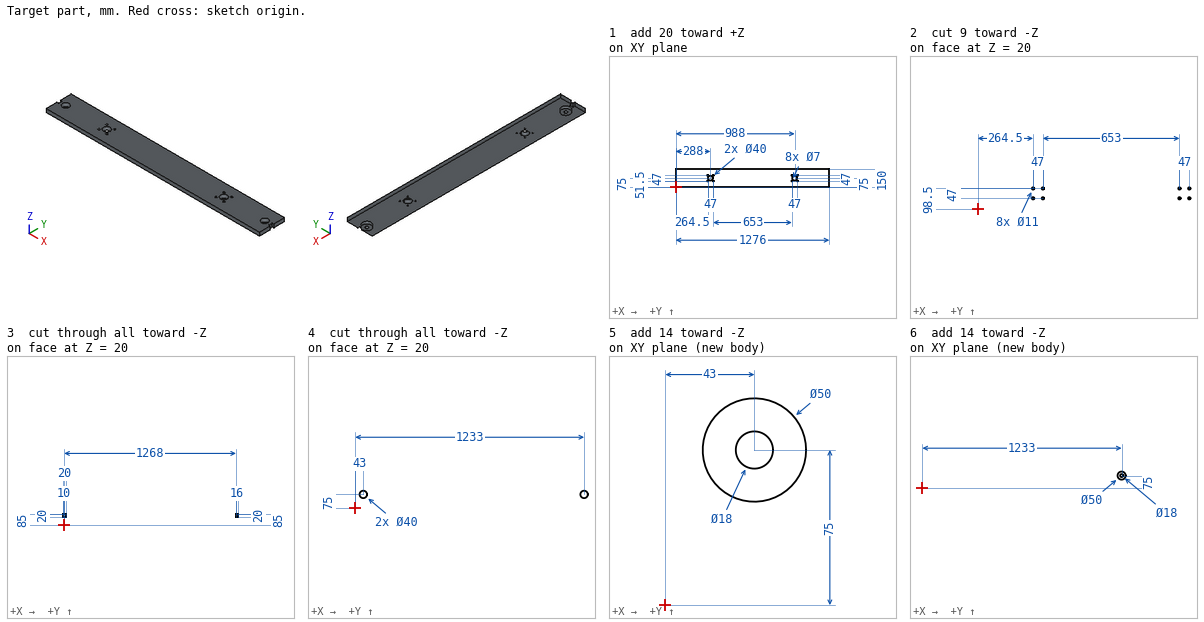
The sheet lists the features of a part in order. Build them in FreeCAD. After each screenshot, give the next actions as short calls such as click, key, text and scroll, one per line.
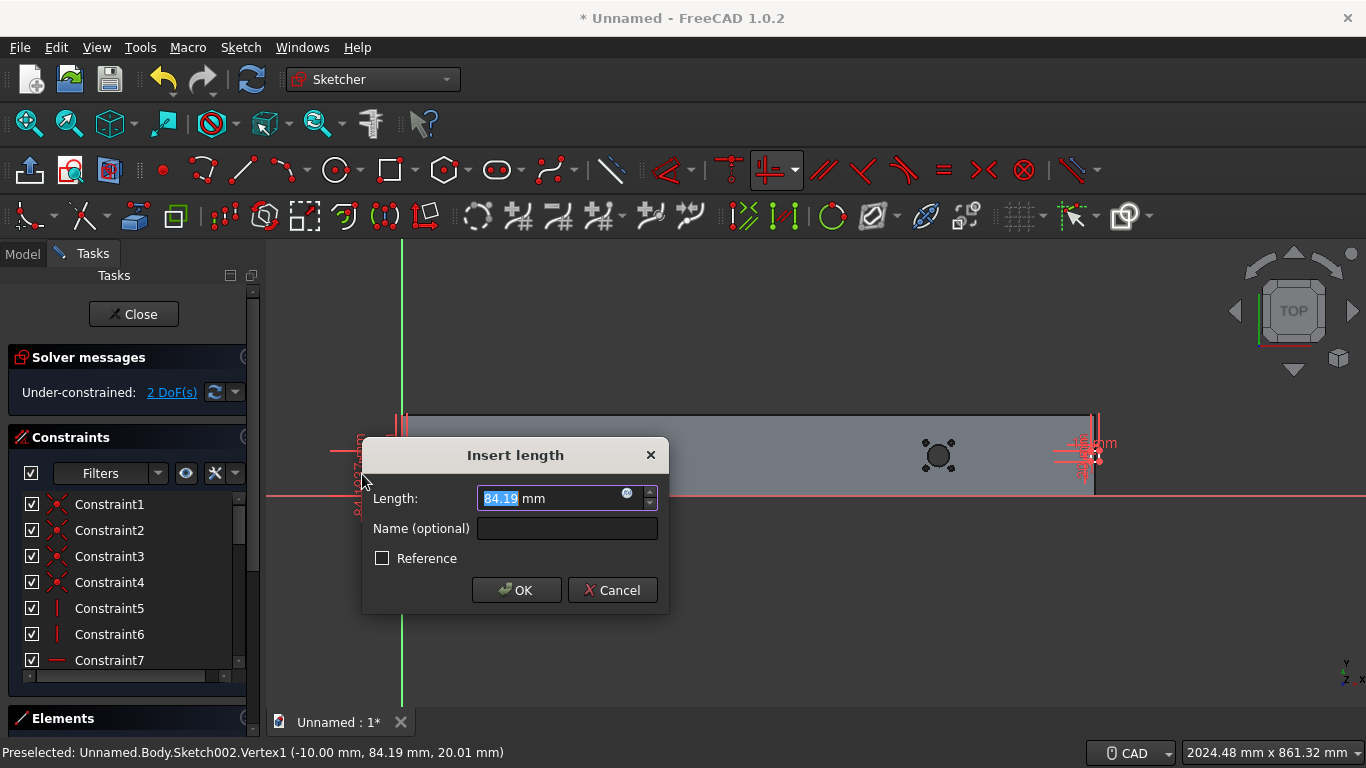
text(85)
key(Return)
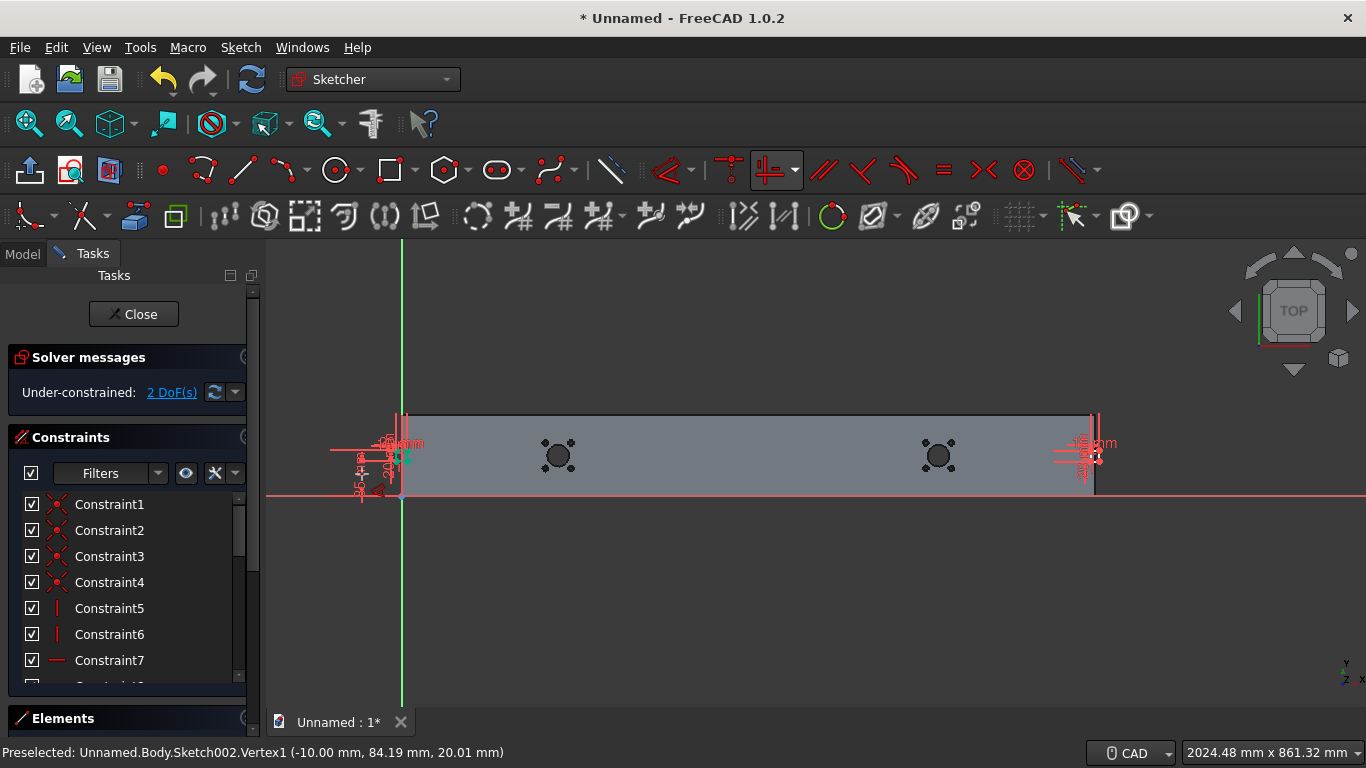
scroll(1091, 451, up, 2)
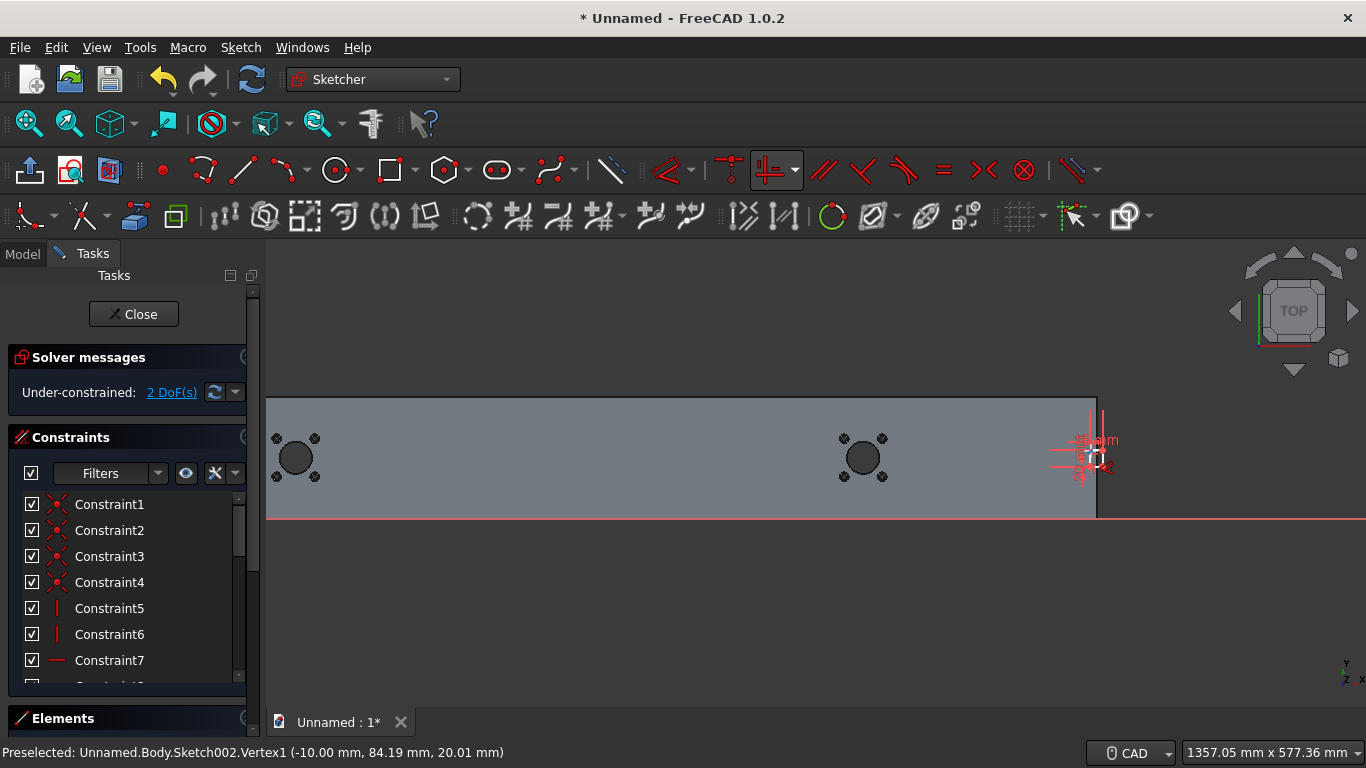
click(1090, 450)
click(1124, 484)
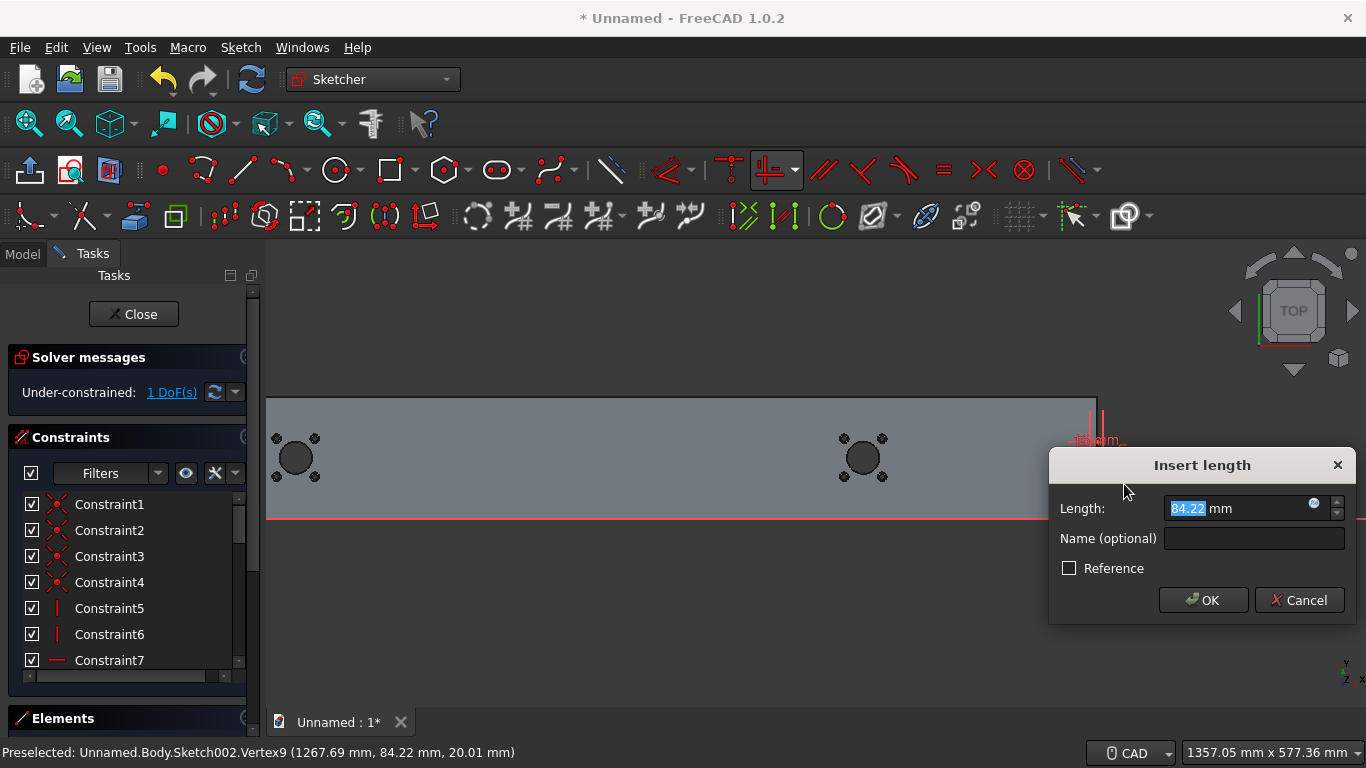
text(85)
key(Return)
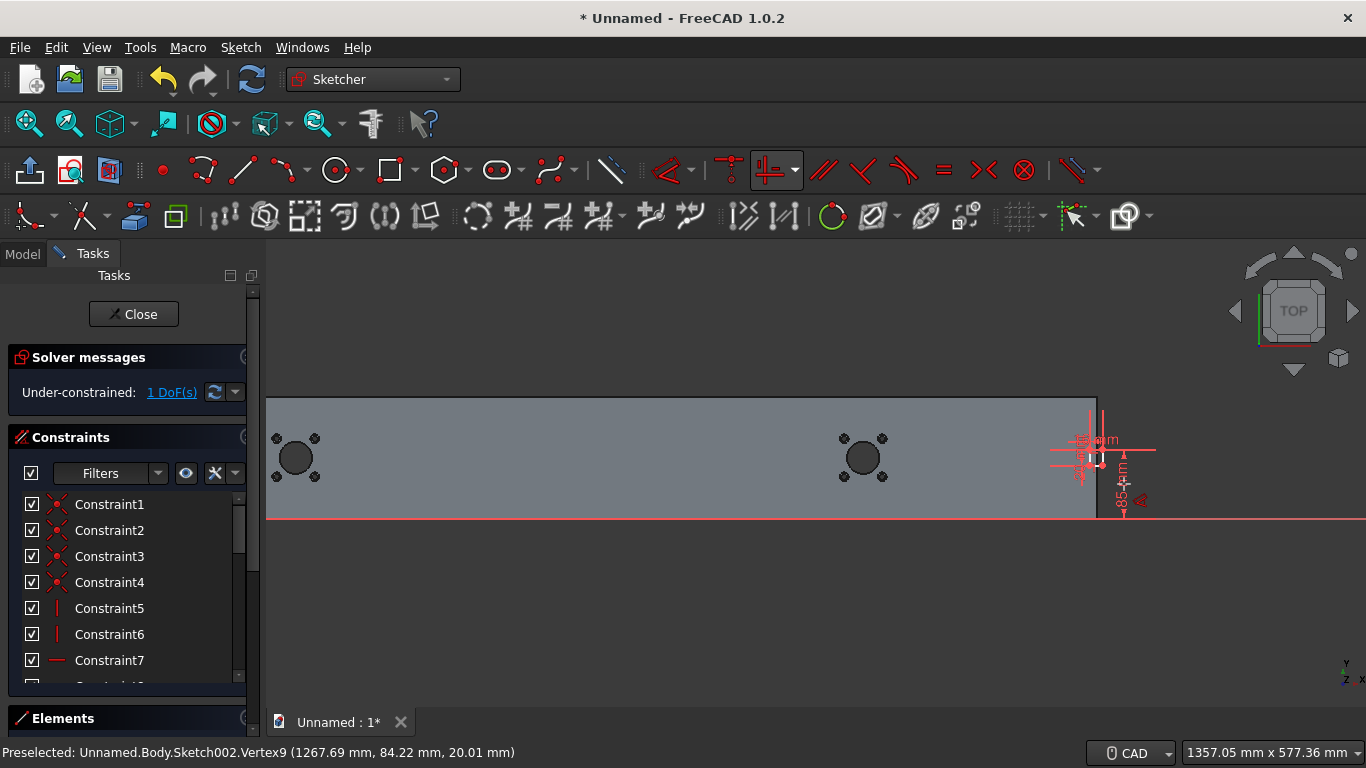
click(1090, 450)
click(692, 553)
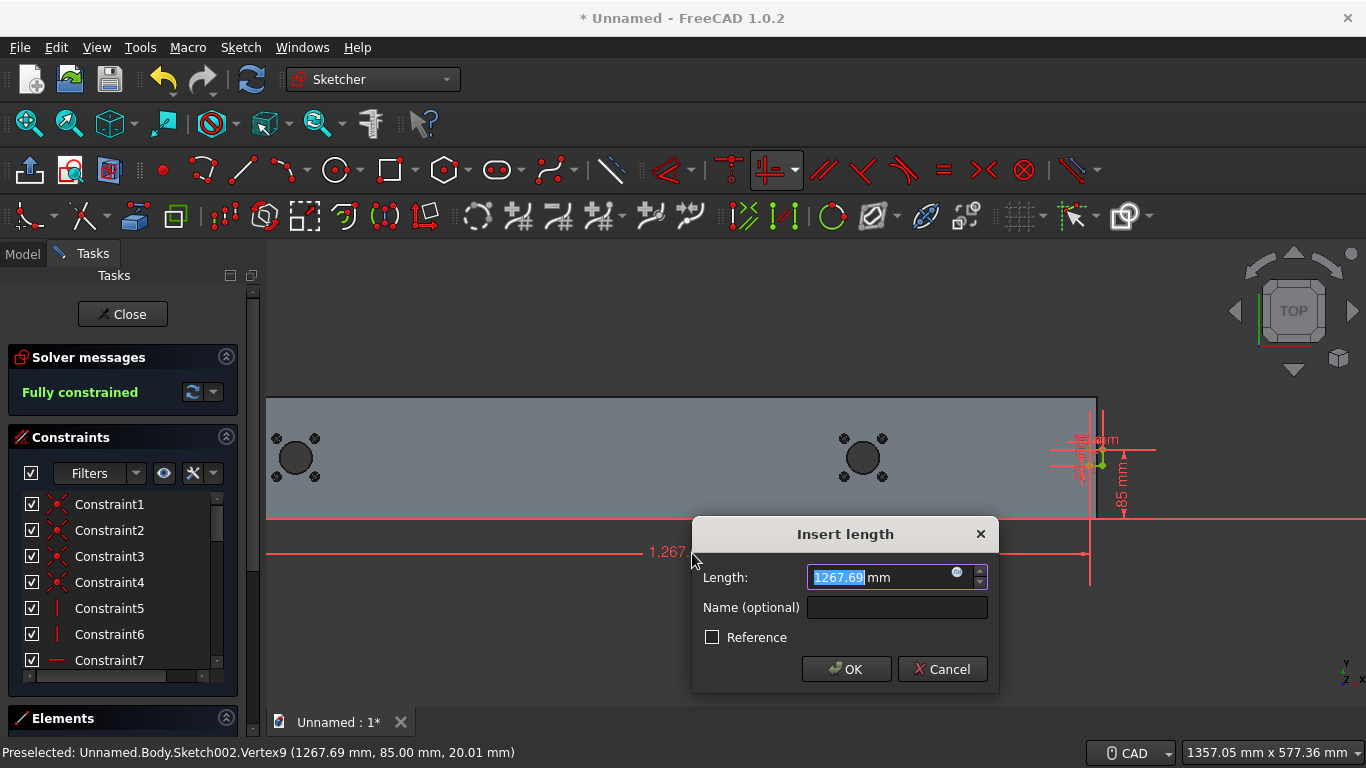
text(1268)
key(Return)
key(Escape)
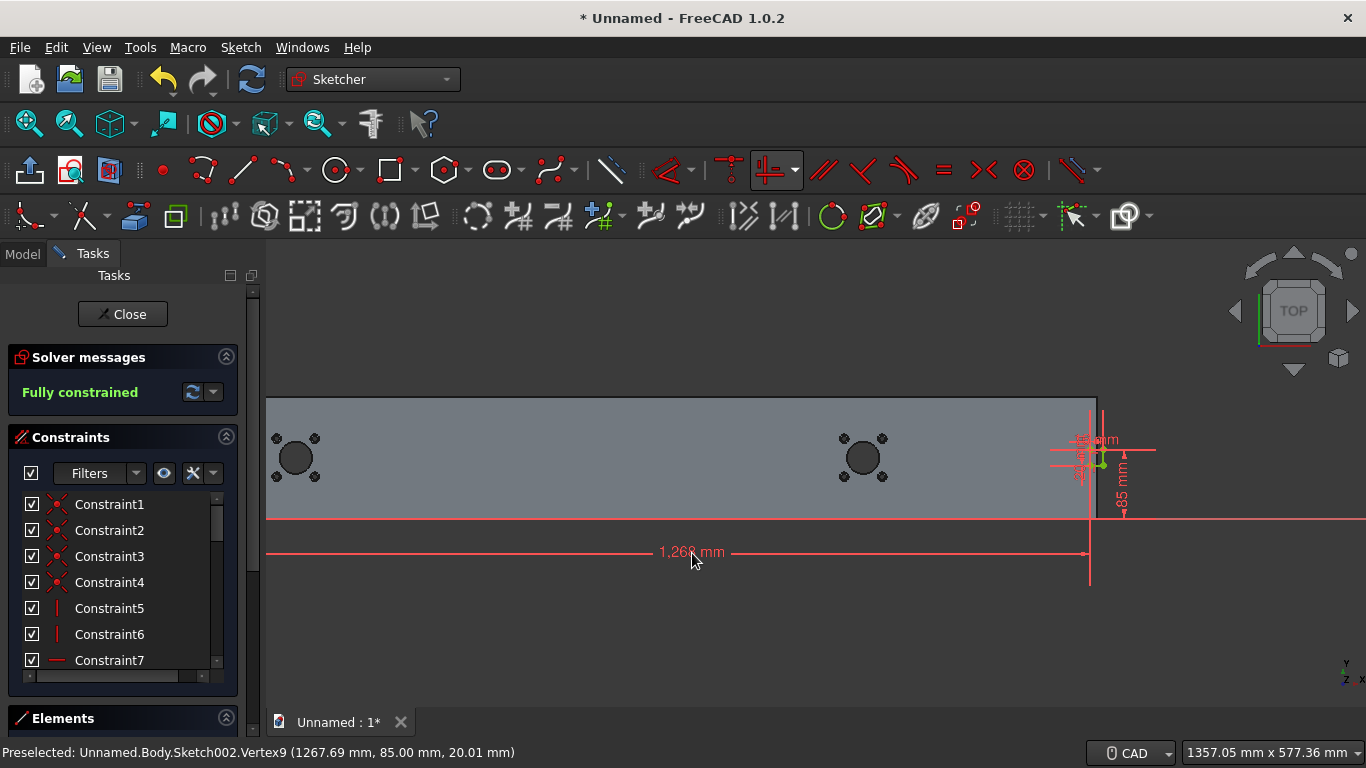
click(123, 314)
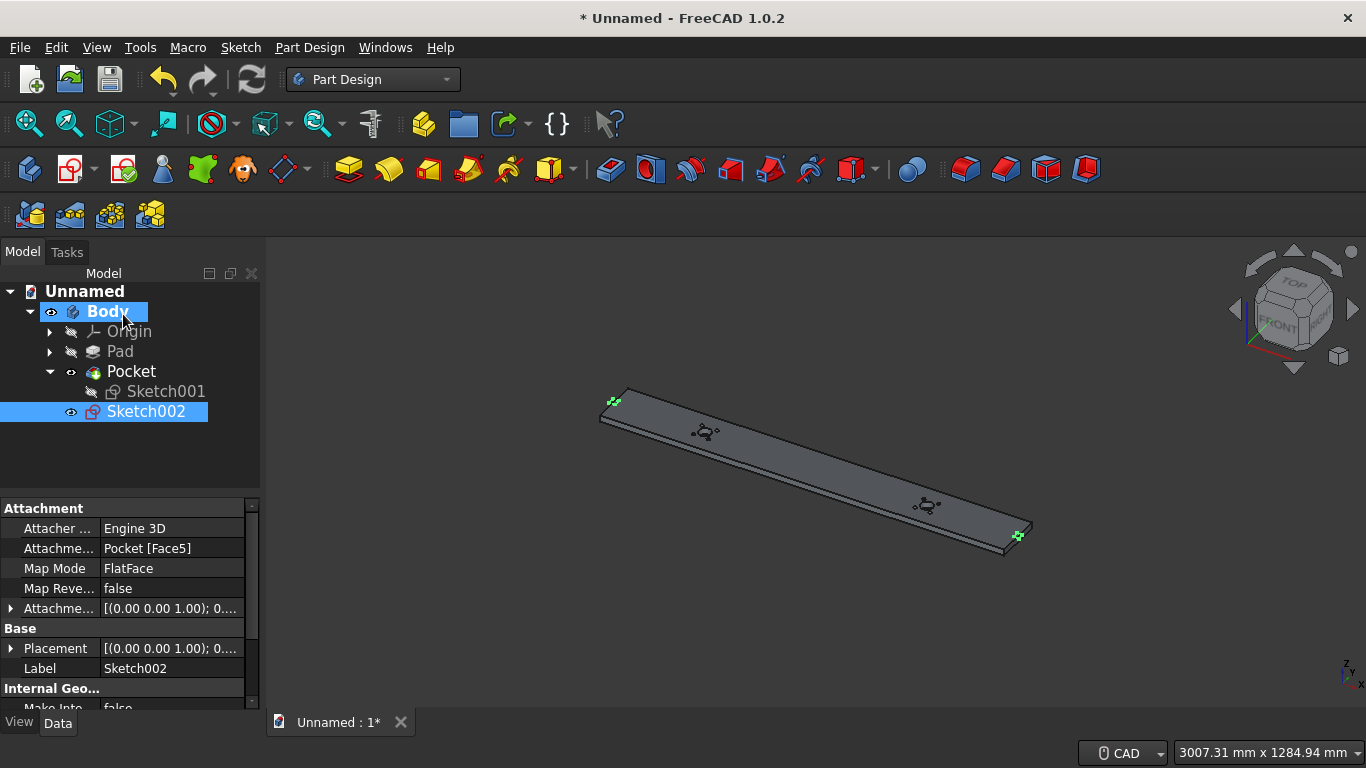
click(612, 170)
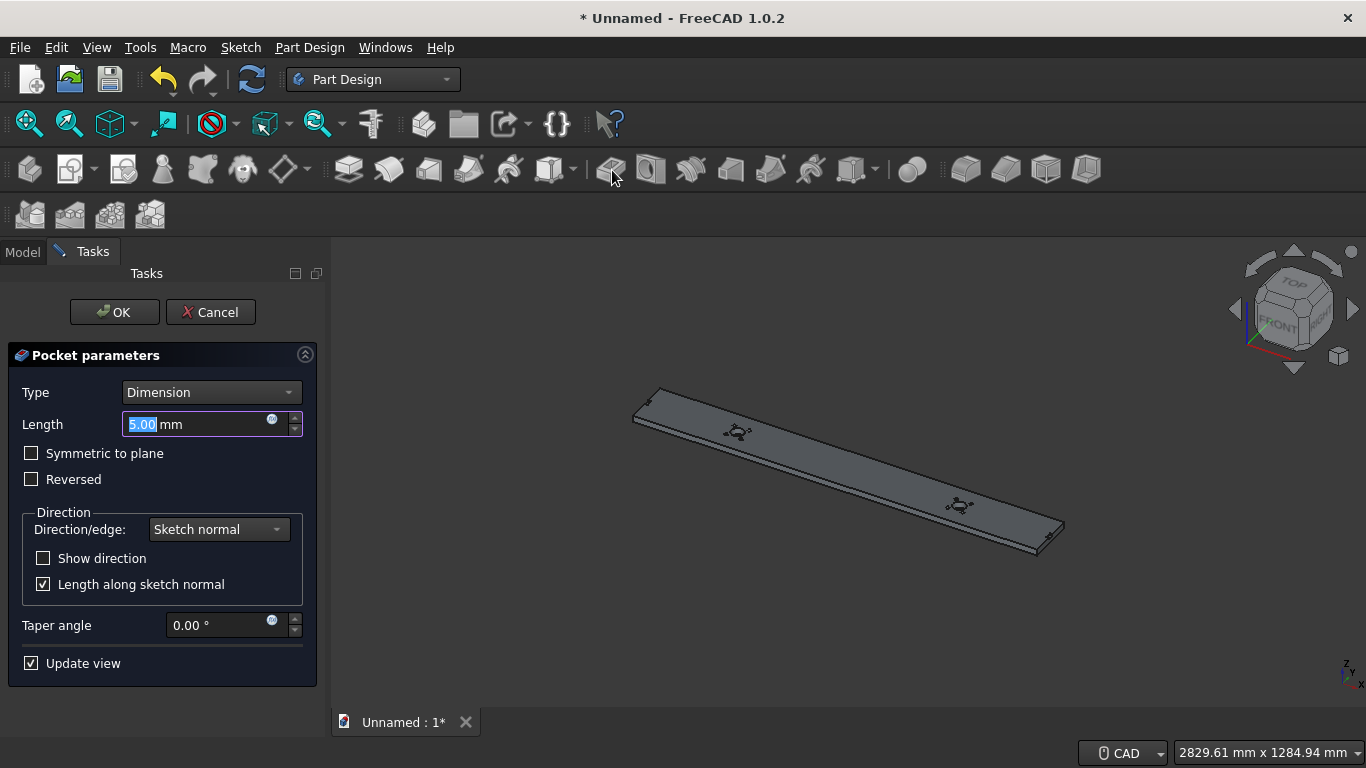
click(212, 392)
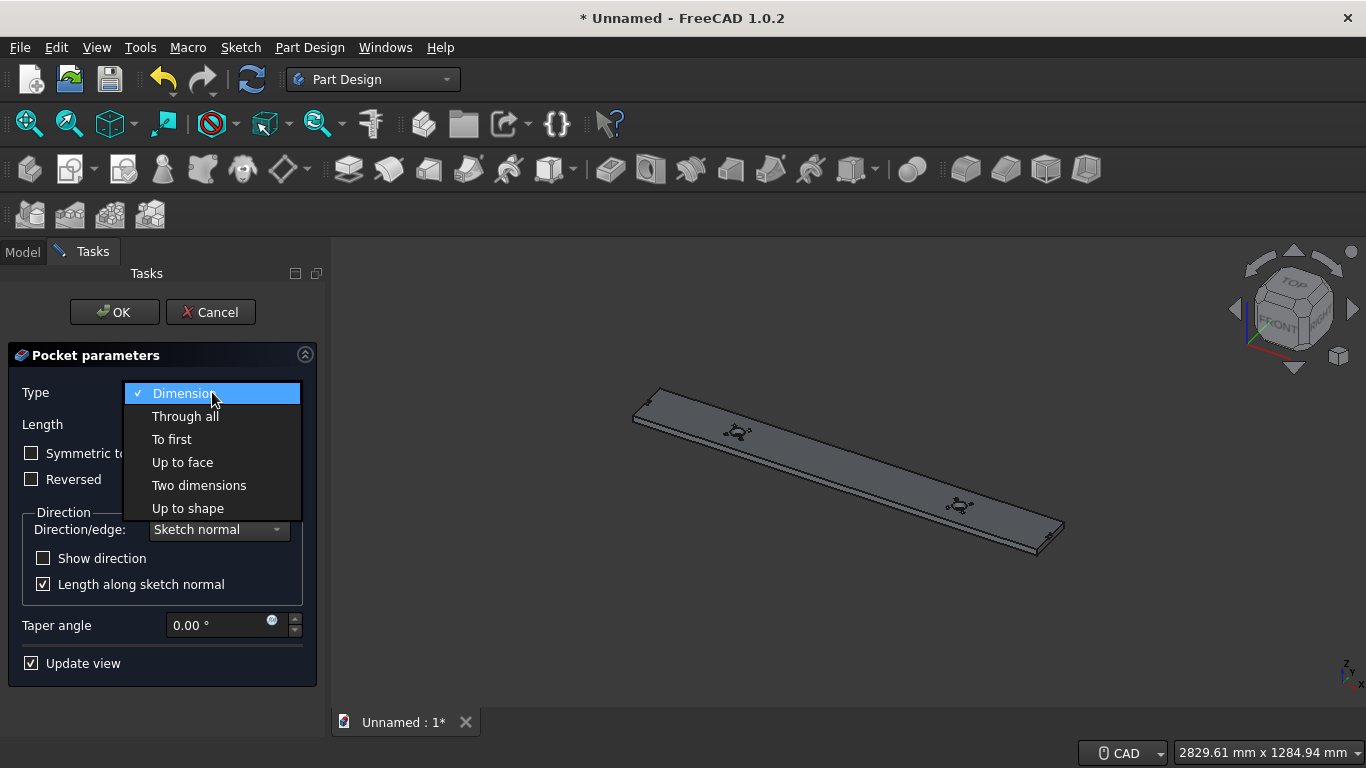
click(212, 416)